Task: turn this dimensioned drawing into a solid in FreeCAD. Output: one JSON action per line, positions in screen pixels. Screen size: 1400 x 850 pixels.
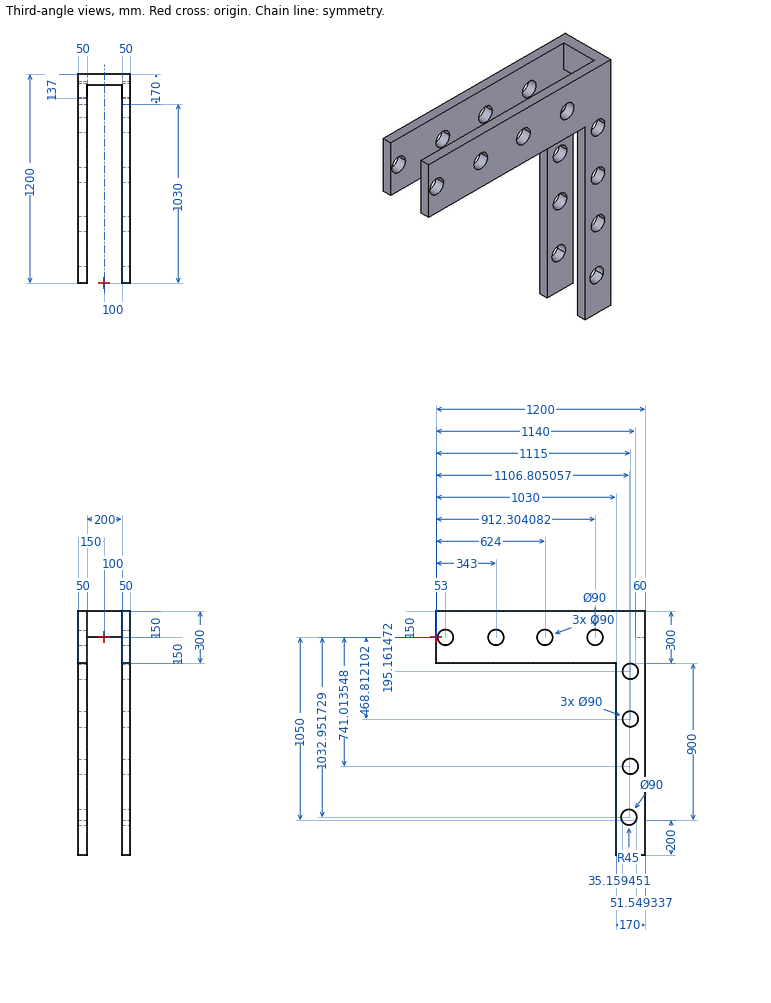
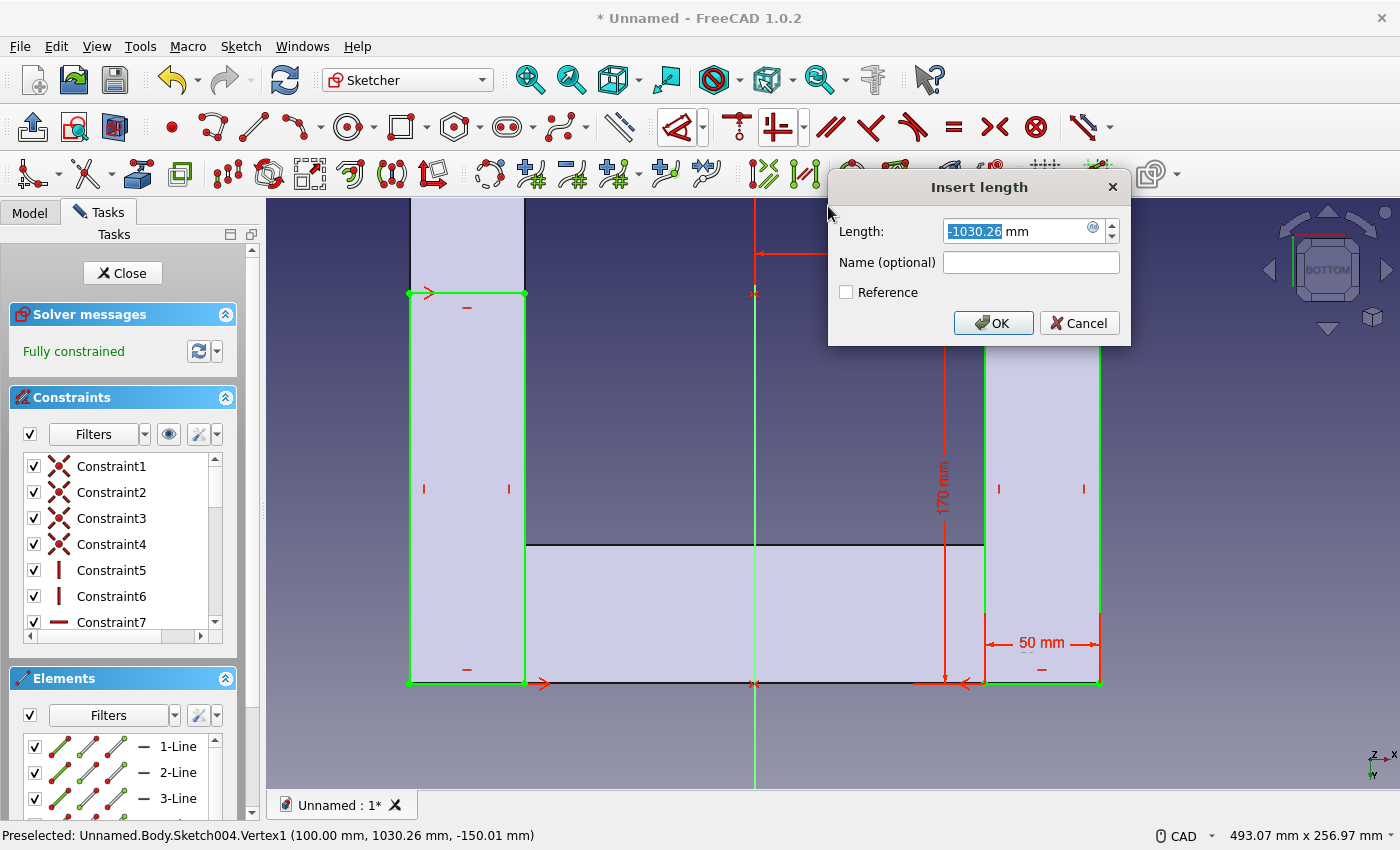
{"action": "type", "text": "-1030"}
{"action": "key", "text": "Return"}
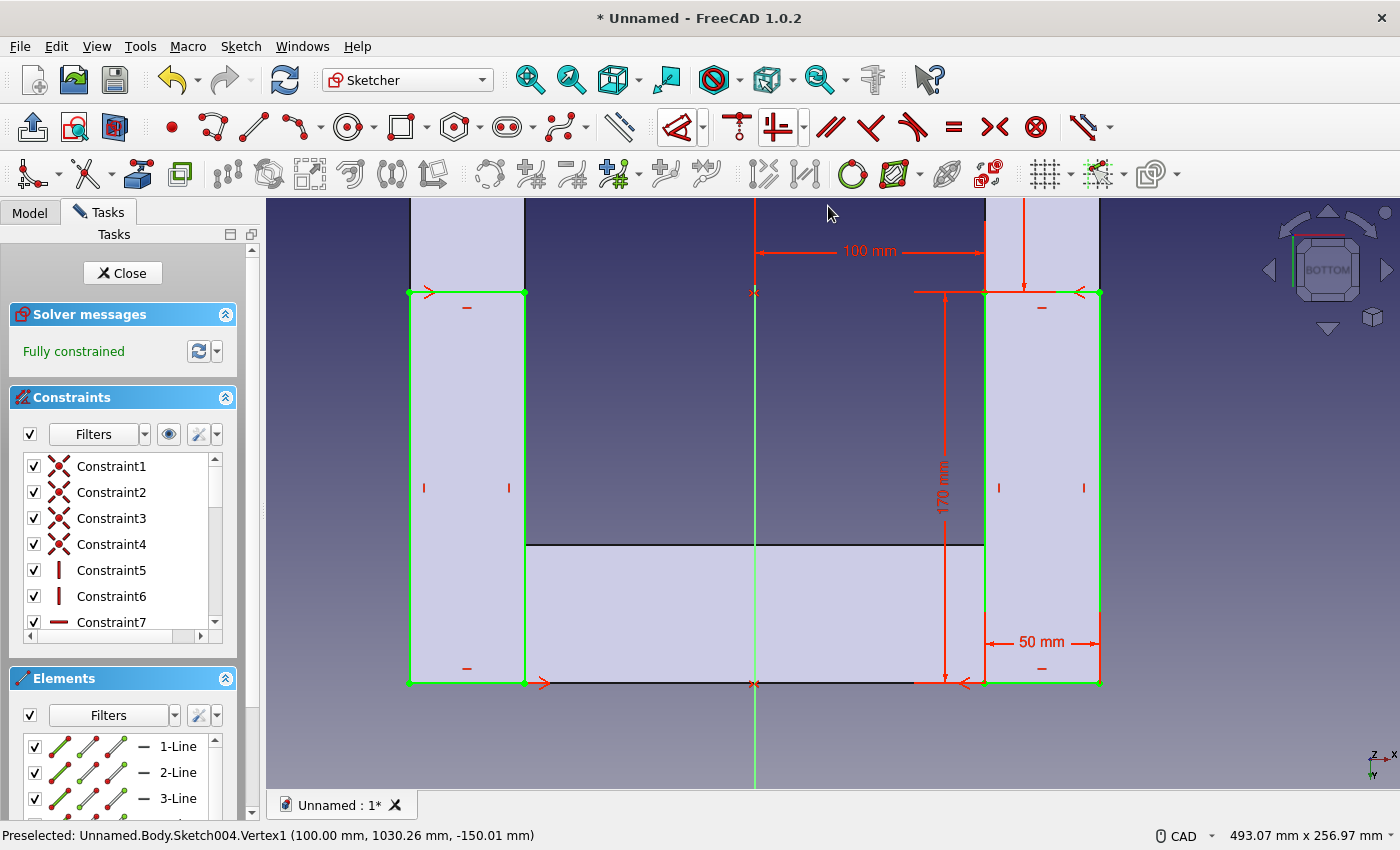
{"action": "left_click", "coordinate": [123, 273]}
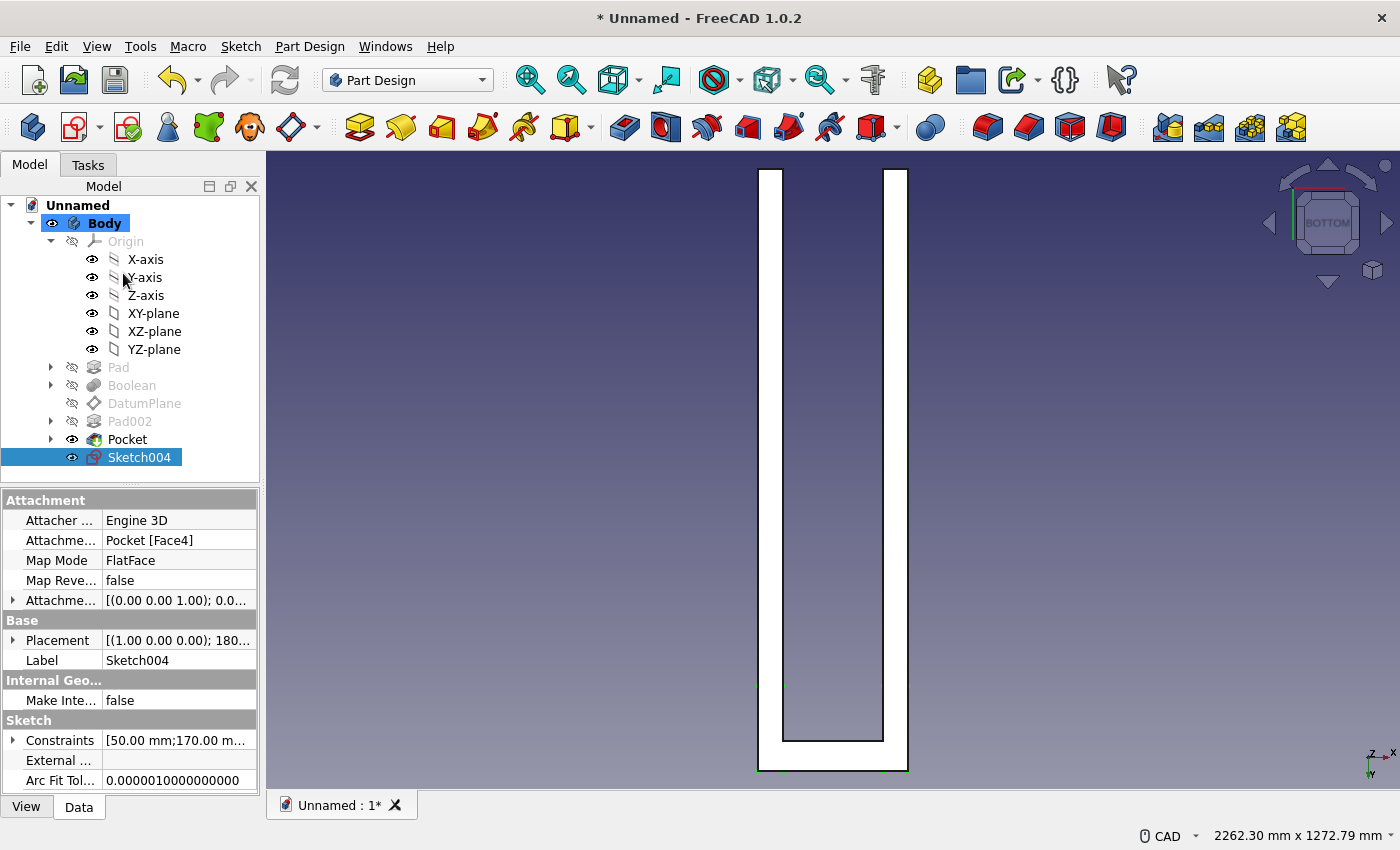
{"action": "left_click", "coordinate": [360, 128]}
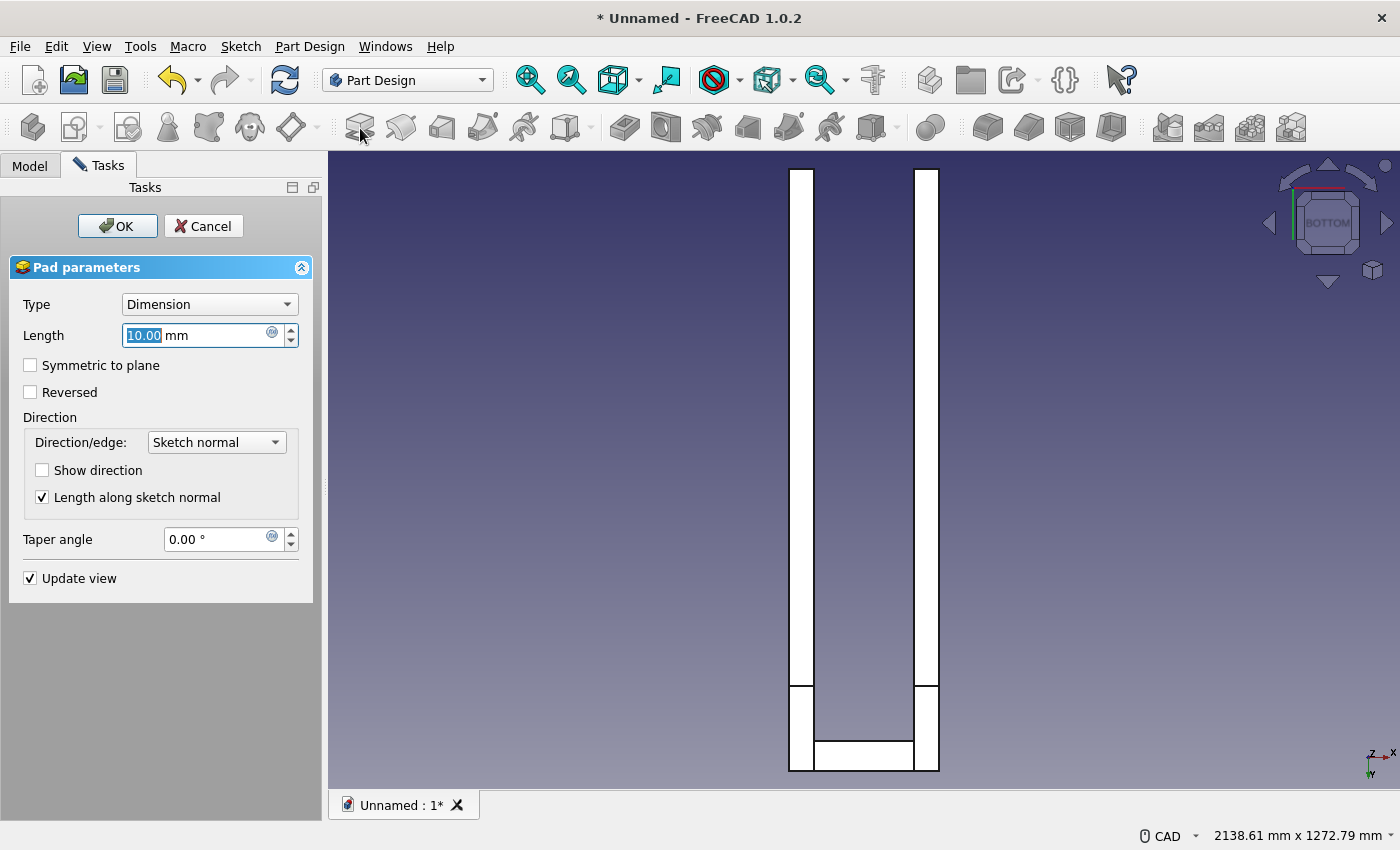
{"action": "type", "text": "900"}
{"action": "key", "text": "Tab"}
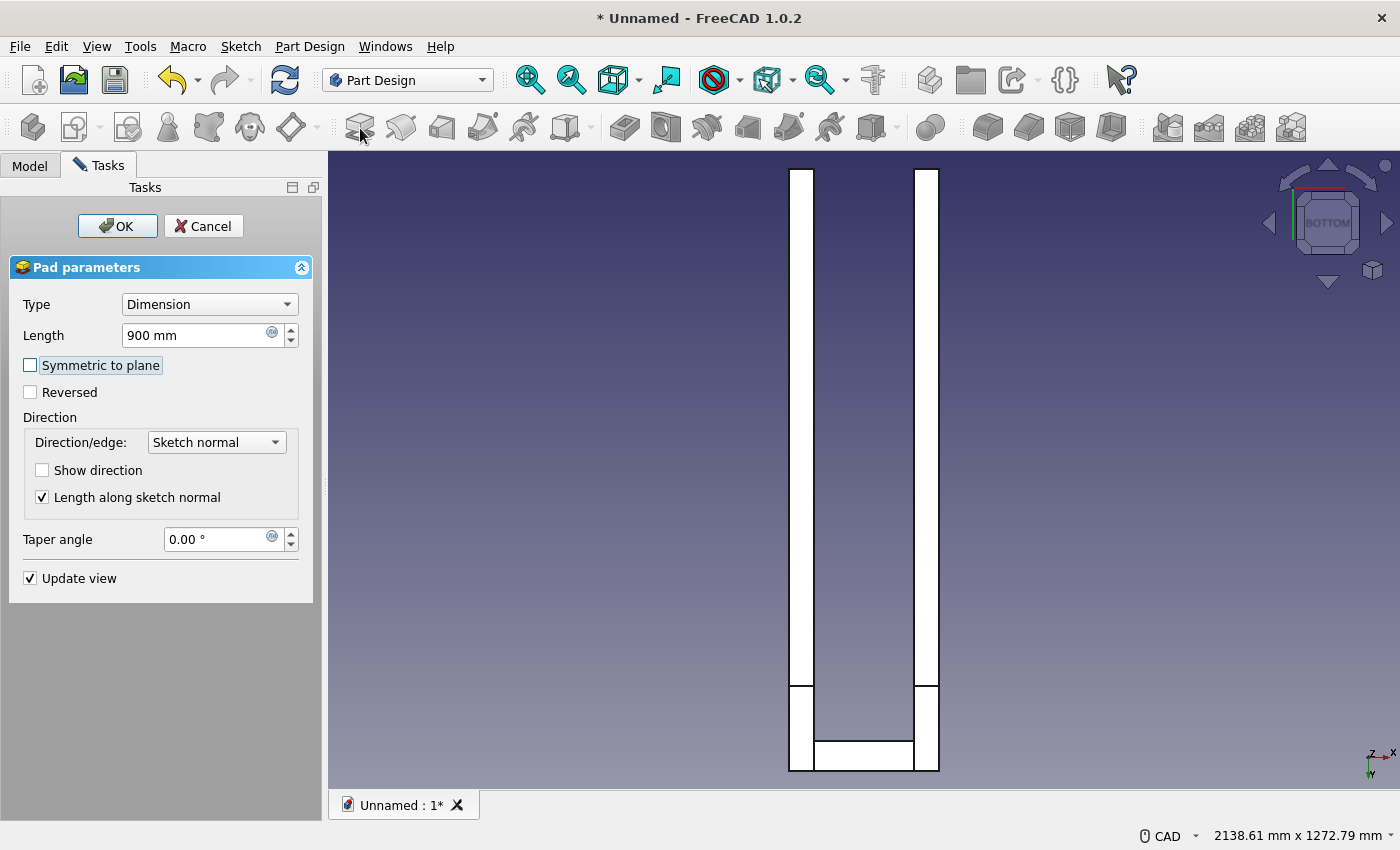
{"action": "left_click", "coordinate": [118, 226]}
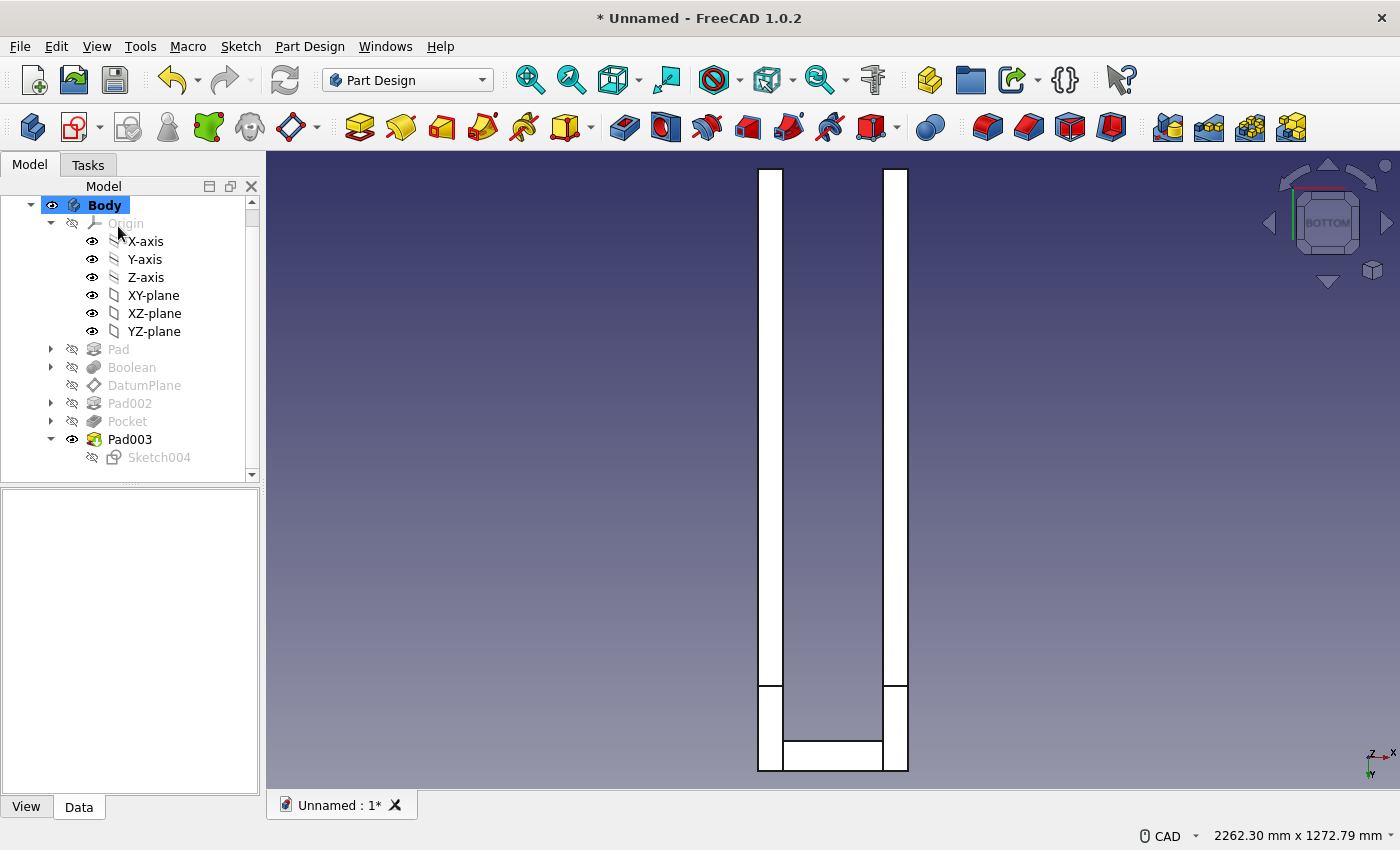
{"action": "key", "text": "0"}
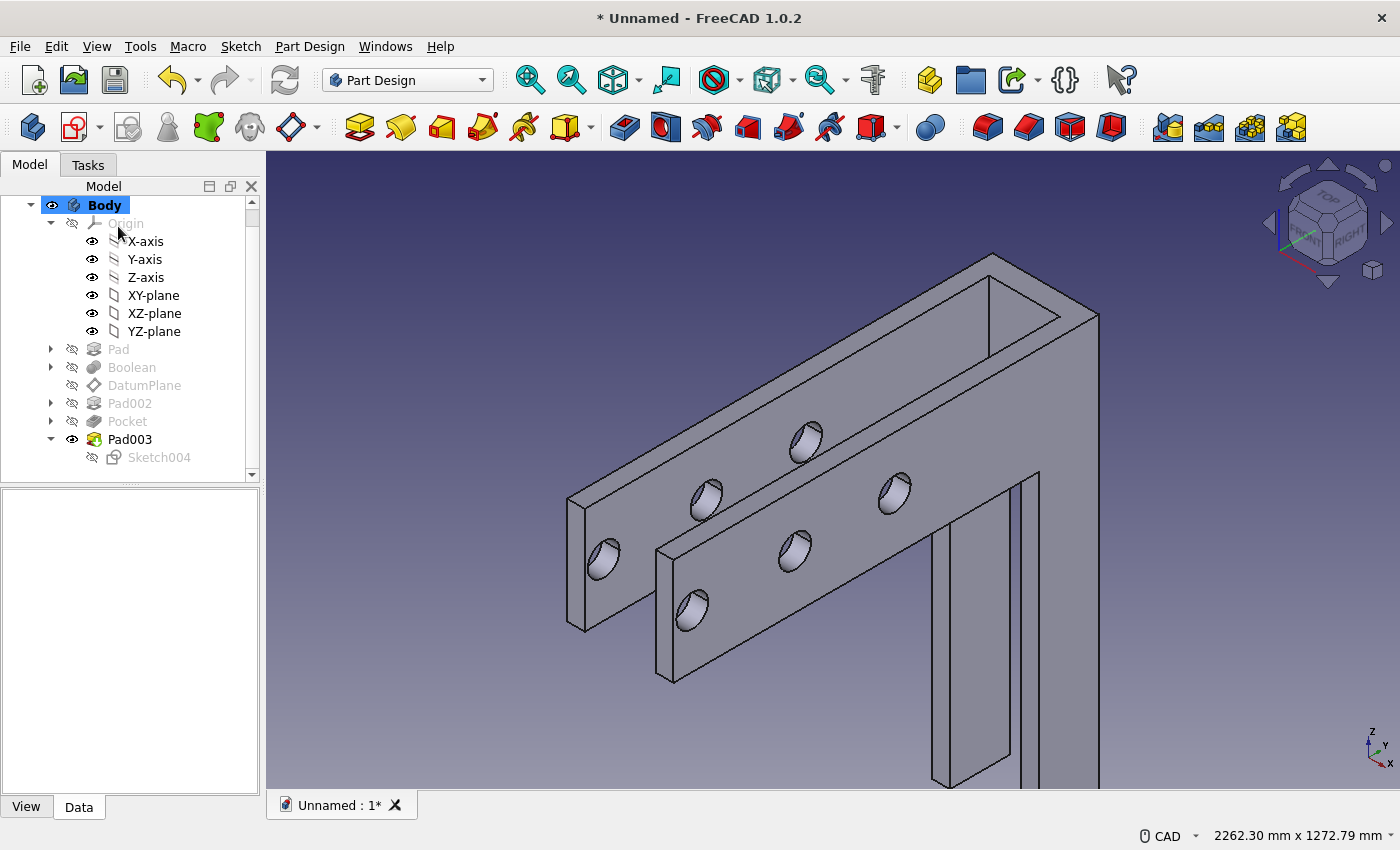
{"action": "left_click", "coordinate": [531, 80]}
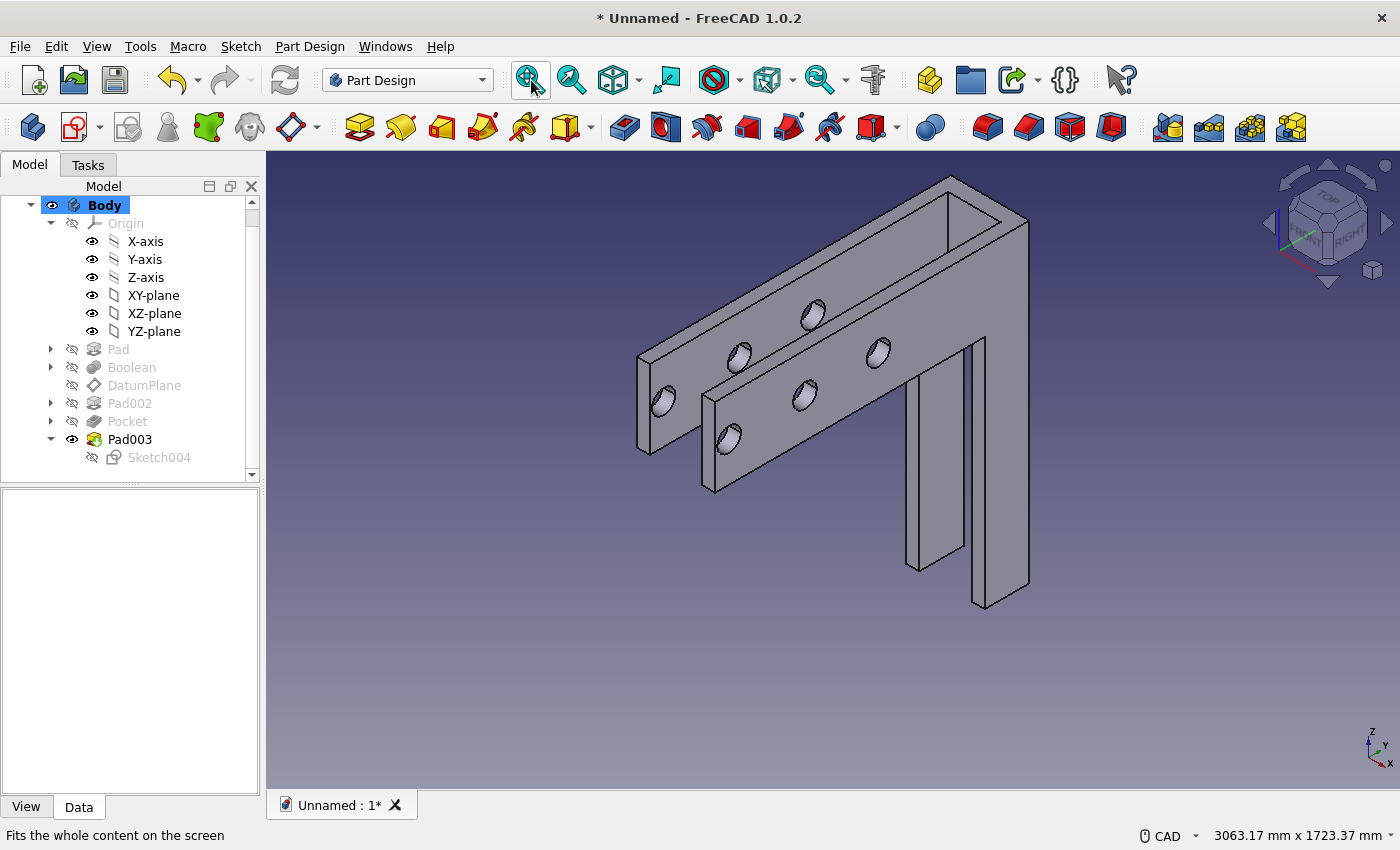
{"action": "left_click", "coordinate": [1007, 310]}